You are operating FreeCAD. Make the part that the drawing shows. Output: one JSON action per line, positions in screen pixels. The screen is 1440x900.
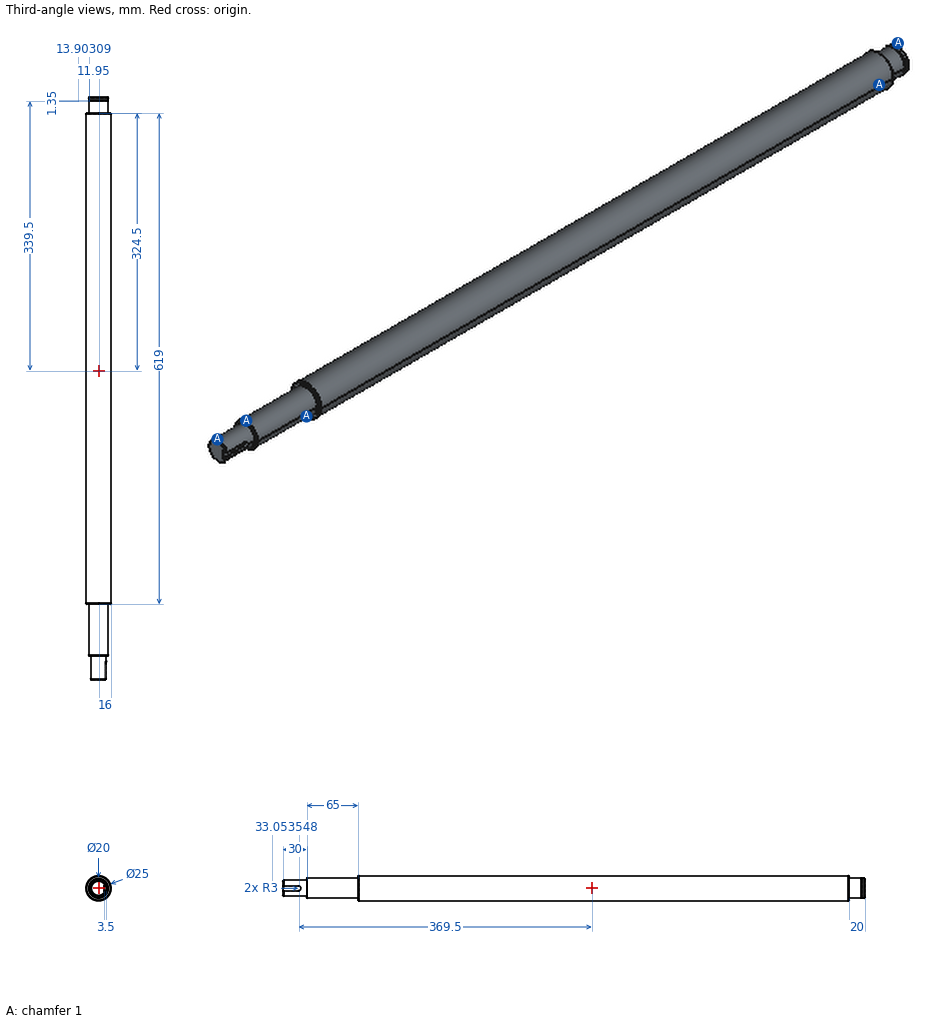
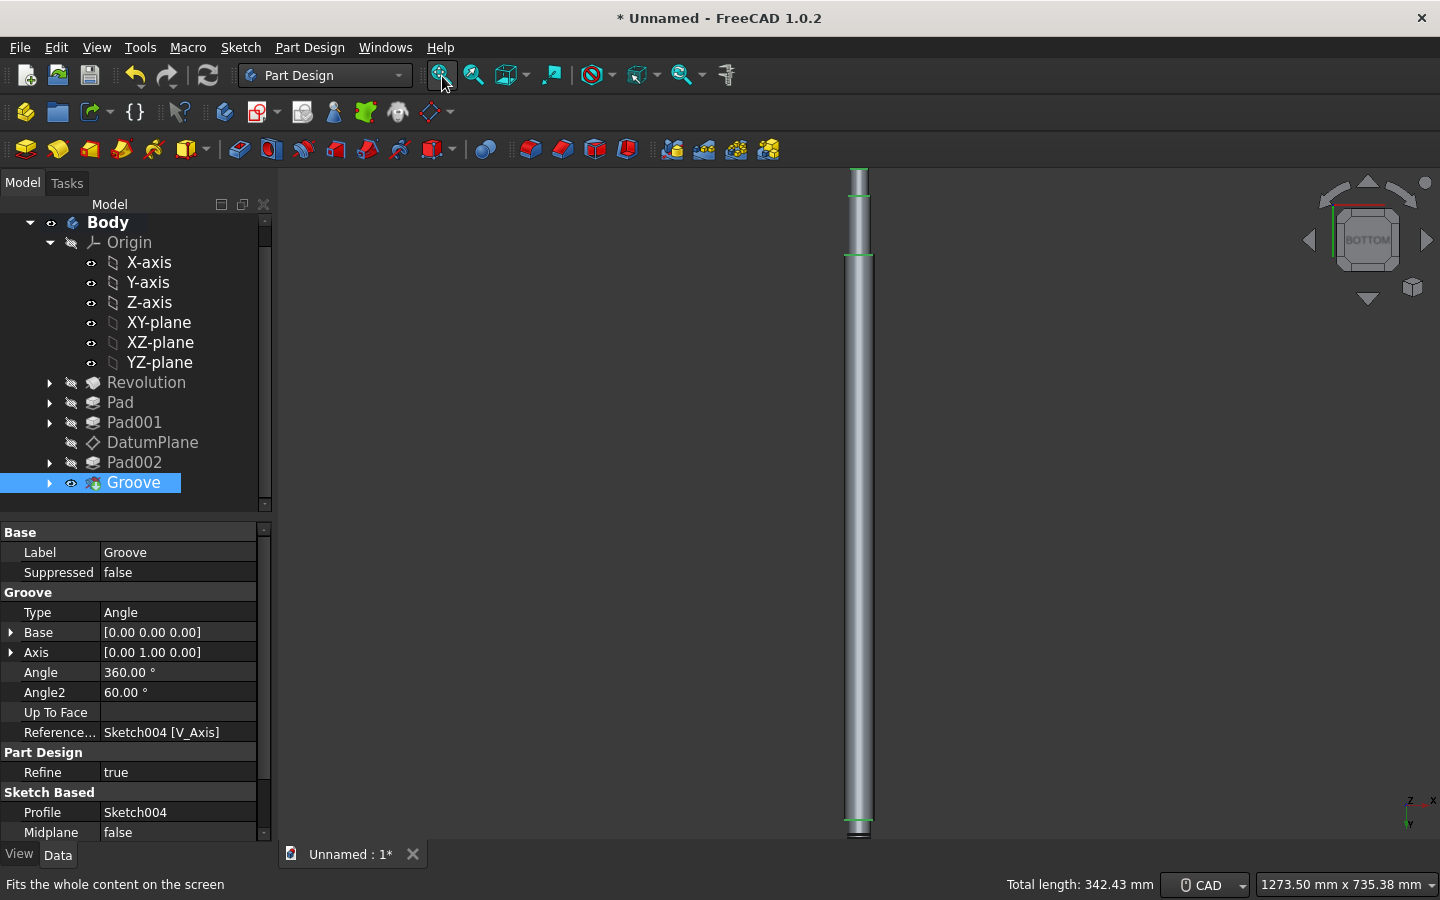
{"action": "key", "text": "4"}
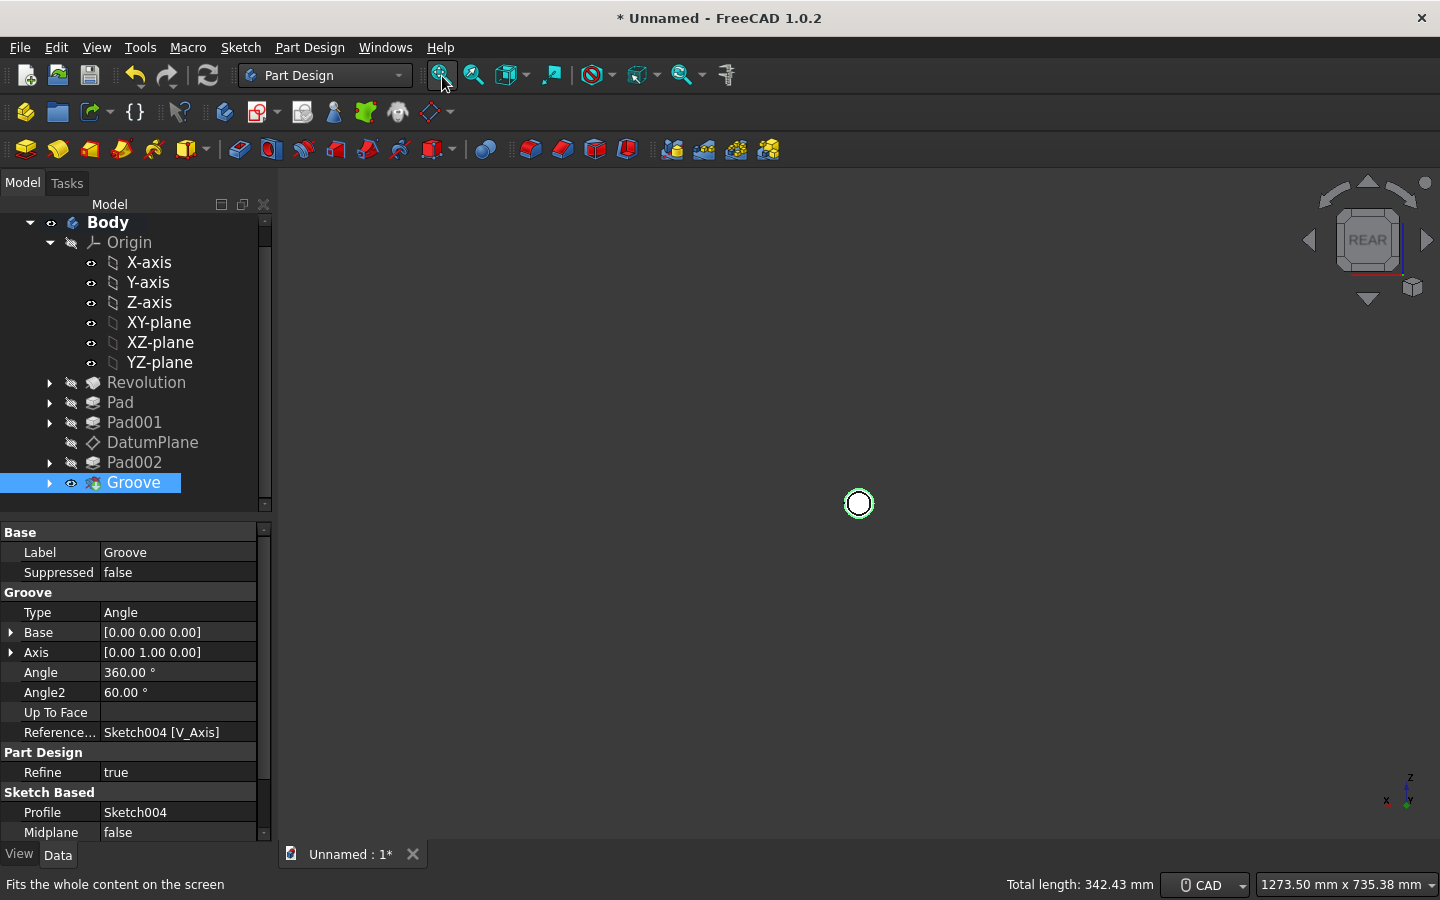
{"action": "left_click", "coordinate": [442, 76]}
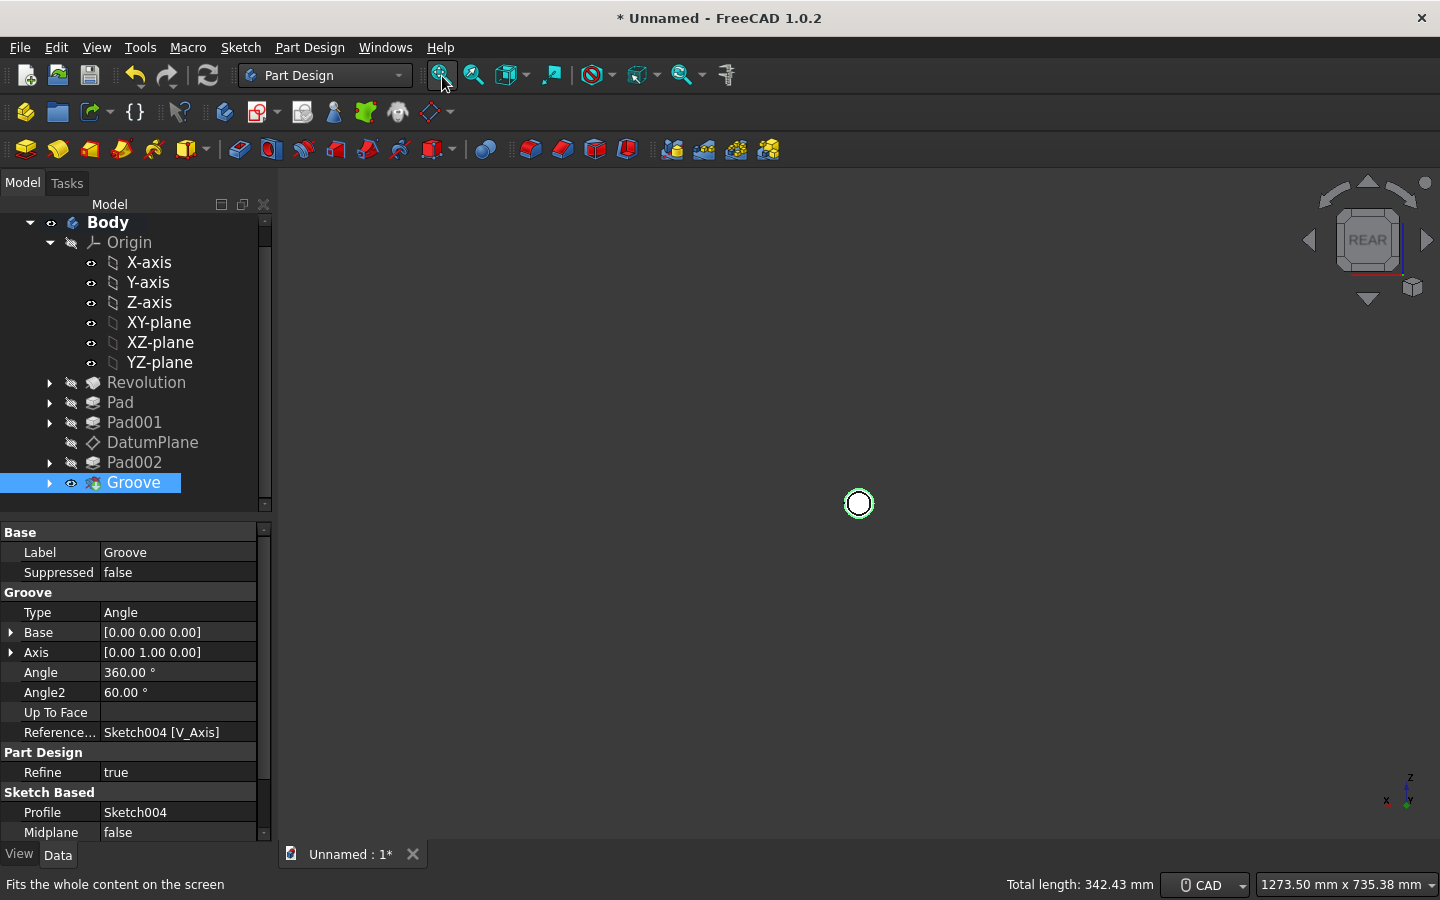
{"action": "left_click", "coordinate": [870, 503], "text": "ctrl"}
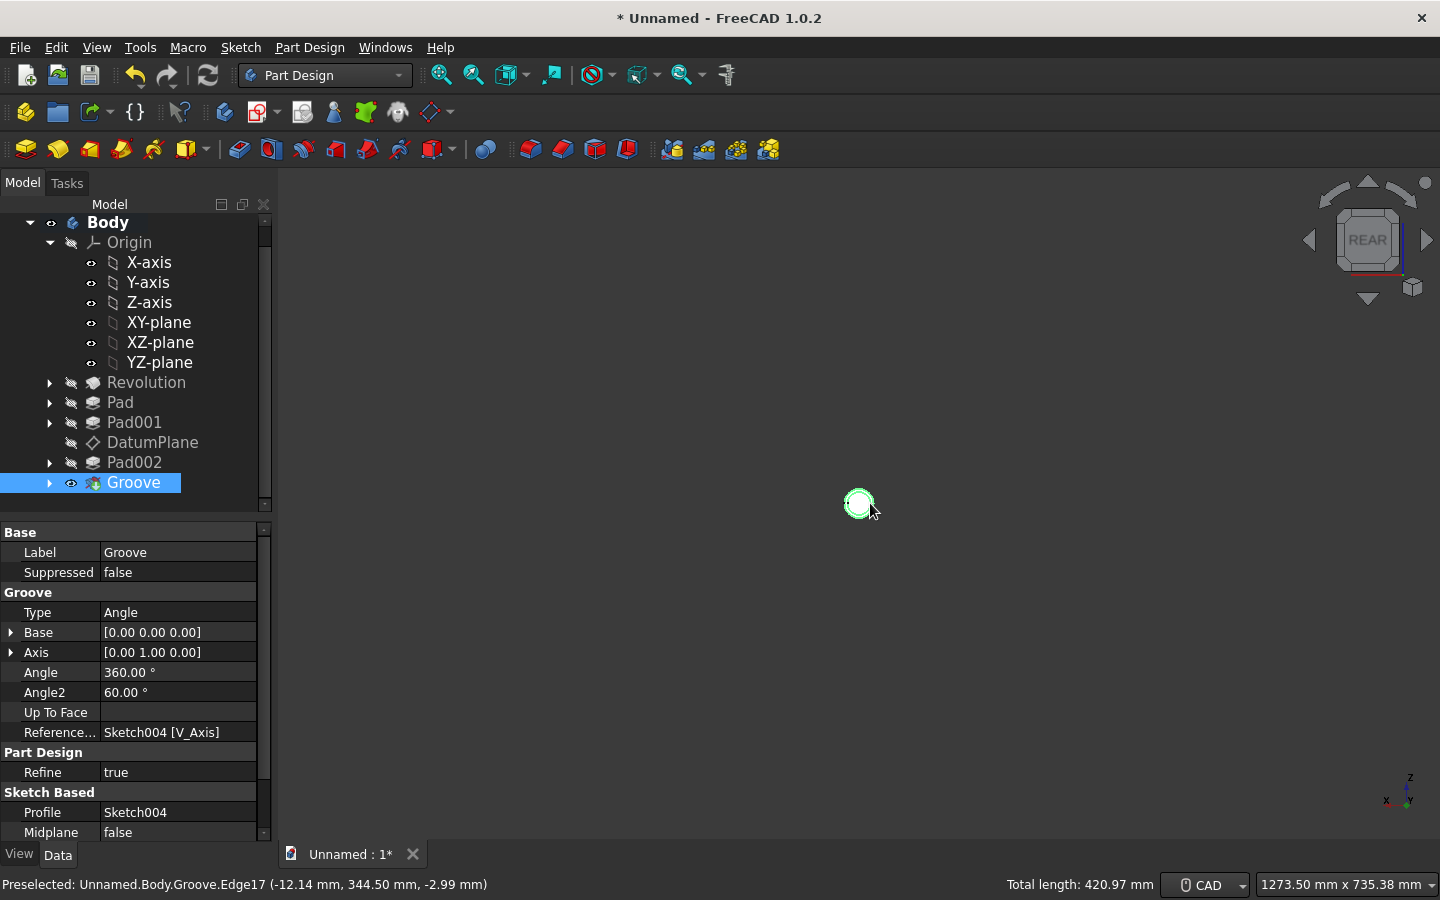
{"action": "left_click", "coordinate": [564, 150]}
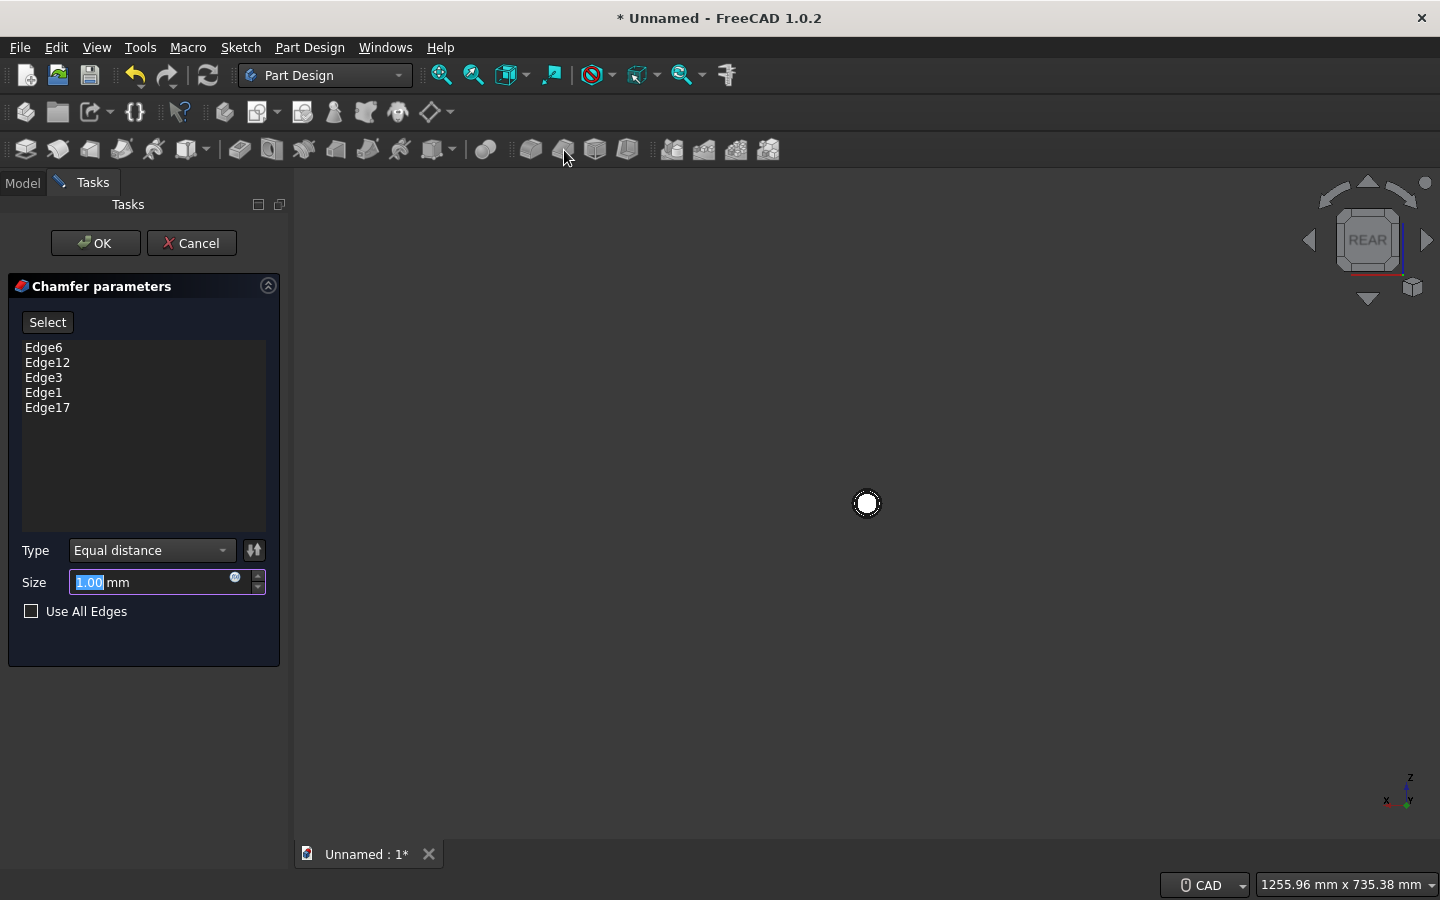
{"action": "type", "text": "1"}
{"action": "key", "text": "Tab"}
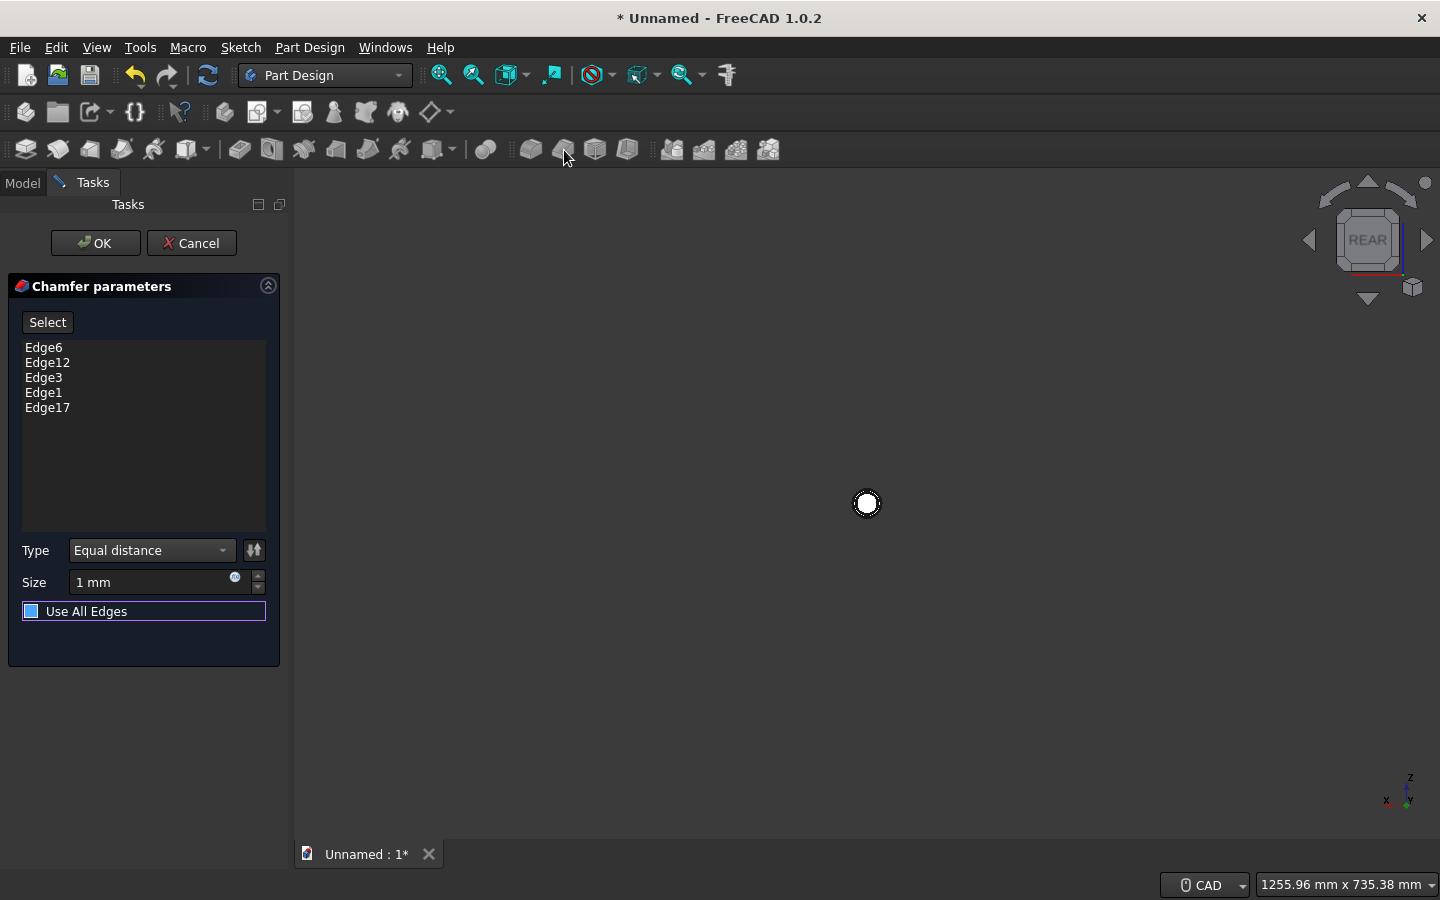
{"action": "left_click", "coordinate": [96, 243]}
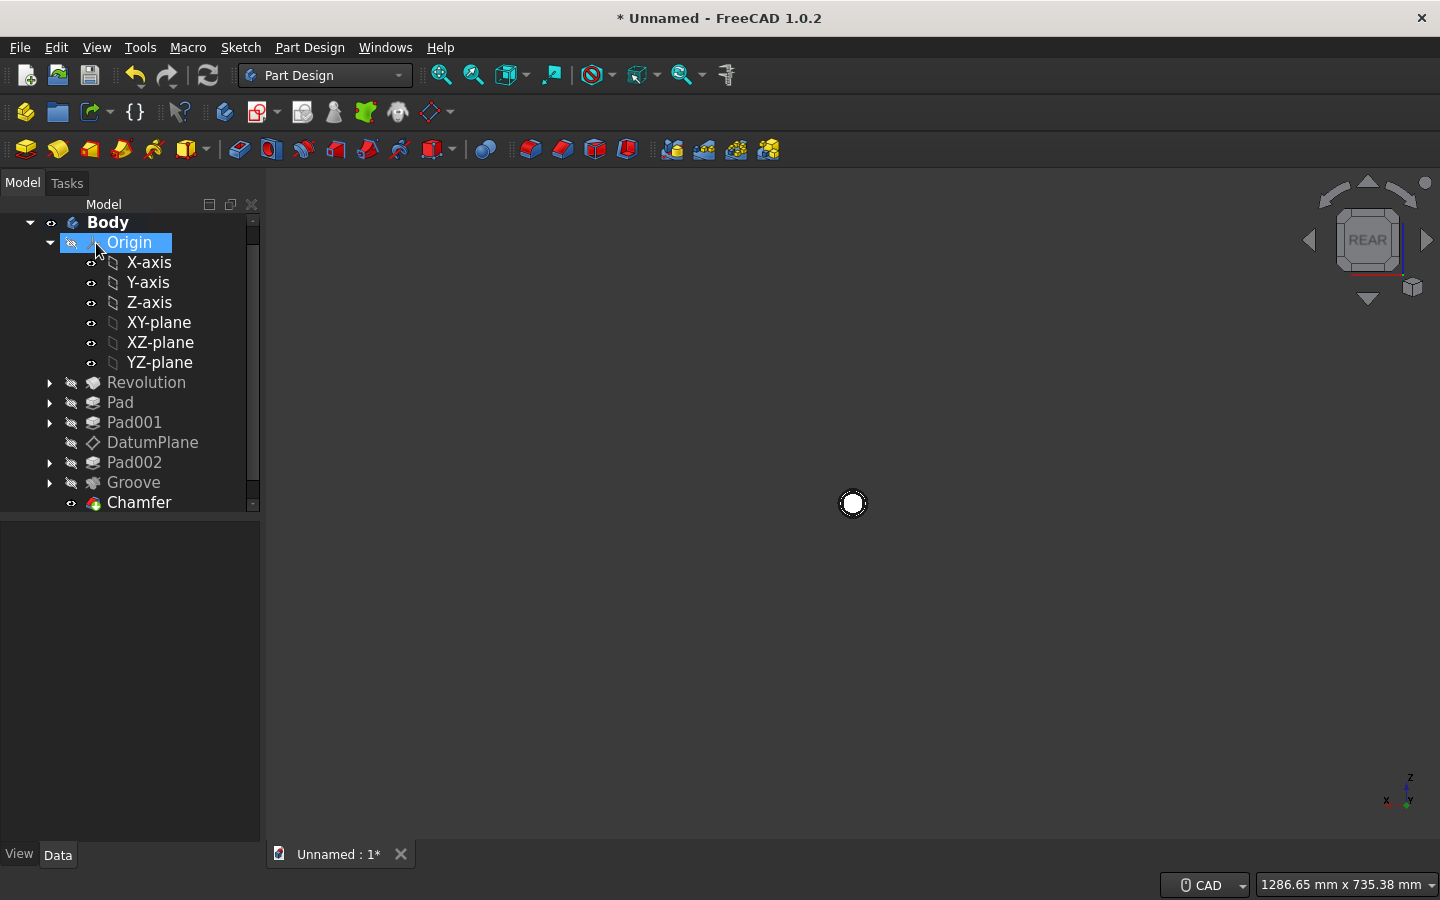
{"action": "left_click", "coordinate": [442, 76]}